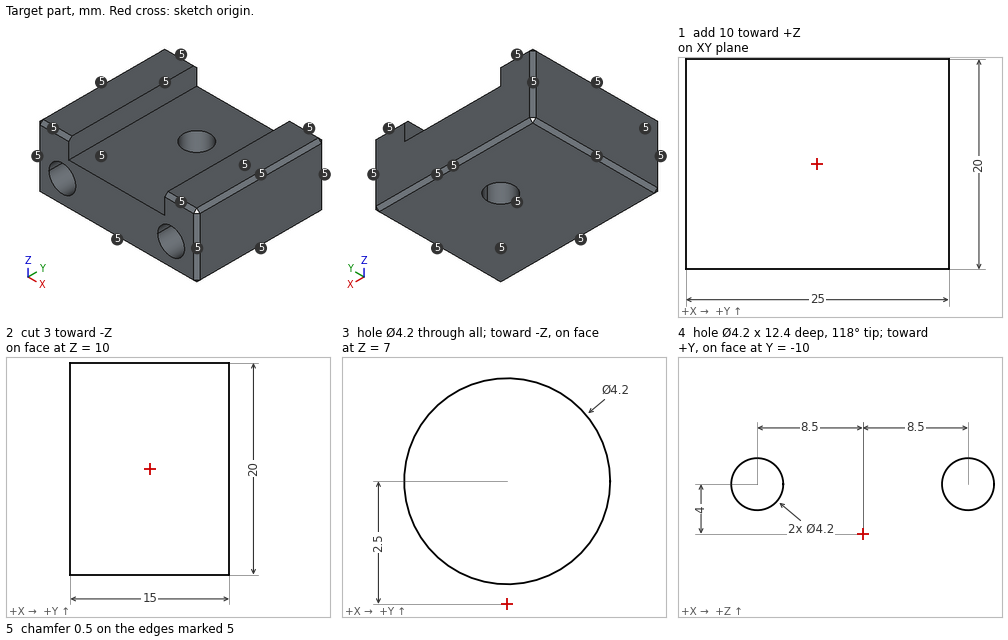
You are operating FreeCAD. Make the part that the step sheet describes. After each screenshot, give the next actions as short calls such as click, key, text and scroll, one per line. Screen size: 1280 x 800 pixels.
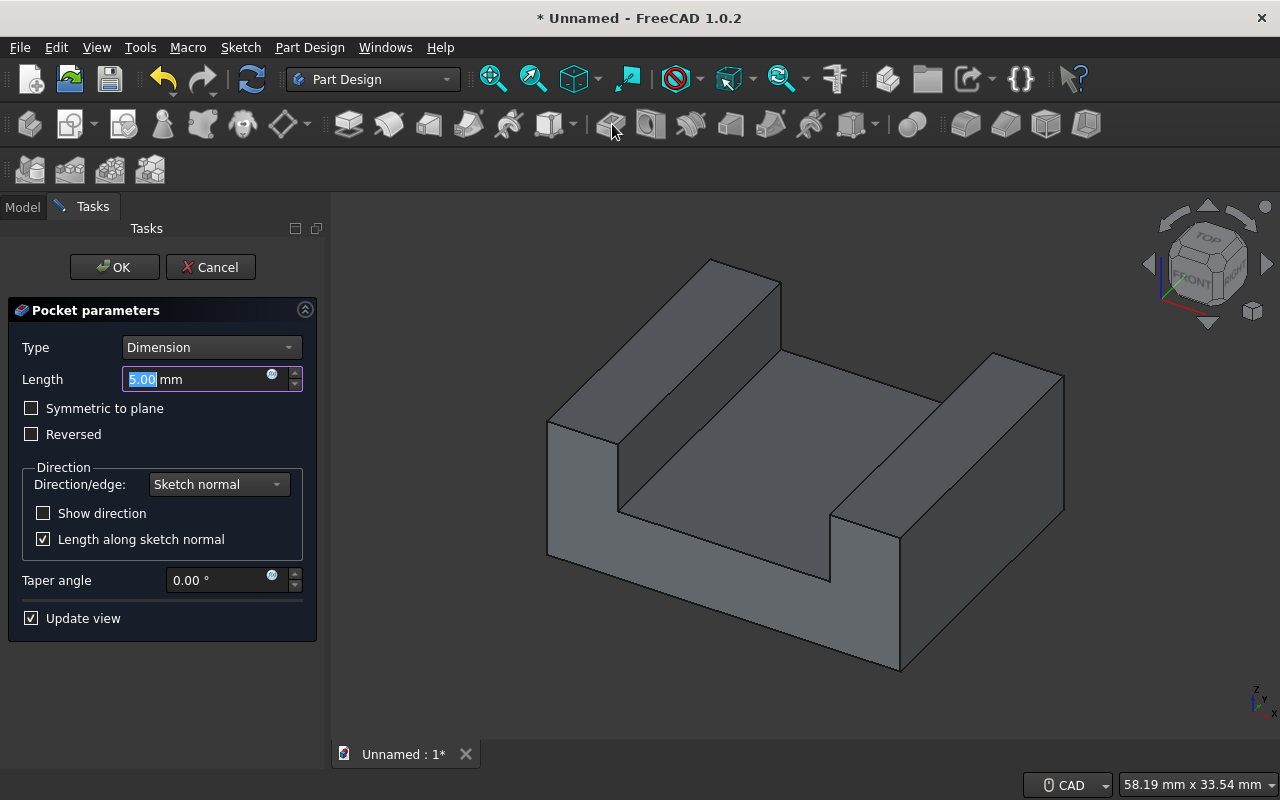
text(3)
key(Tab)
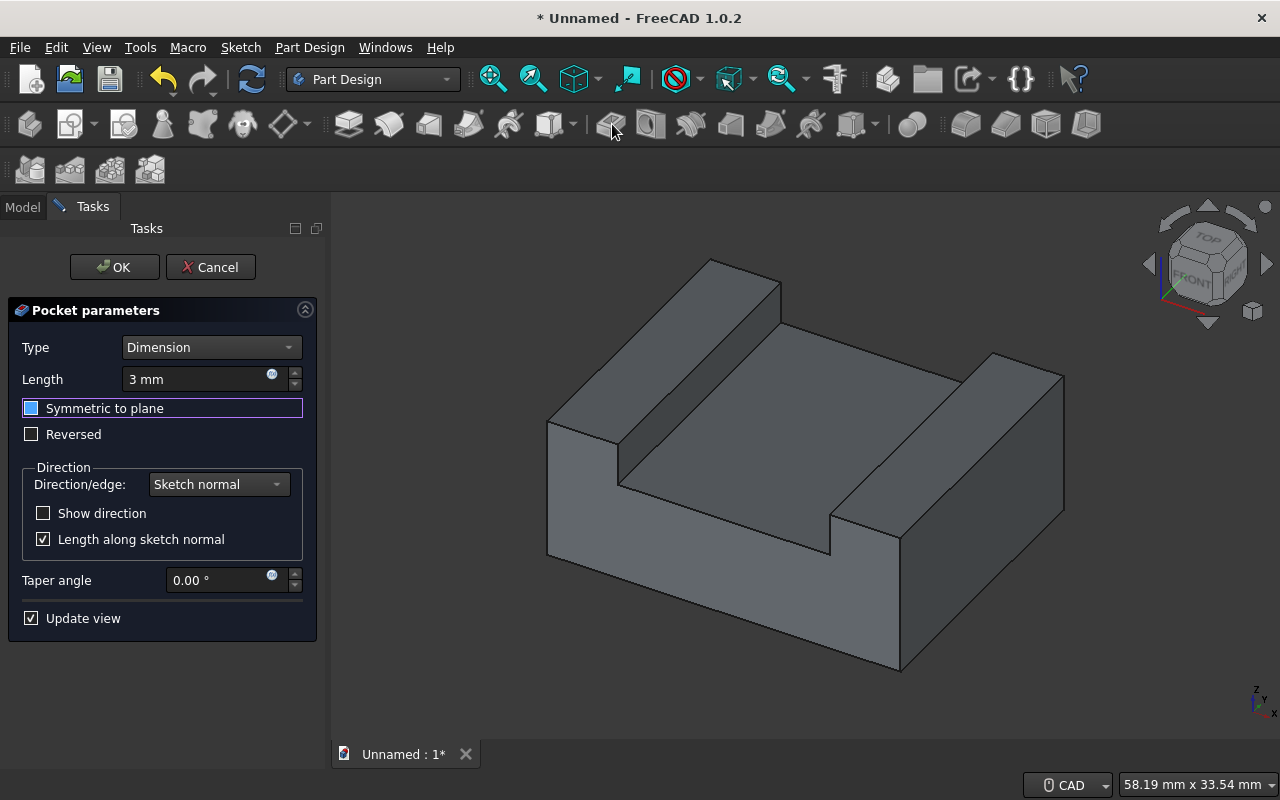
click(115, 267)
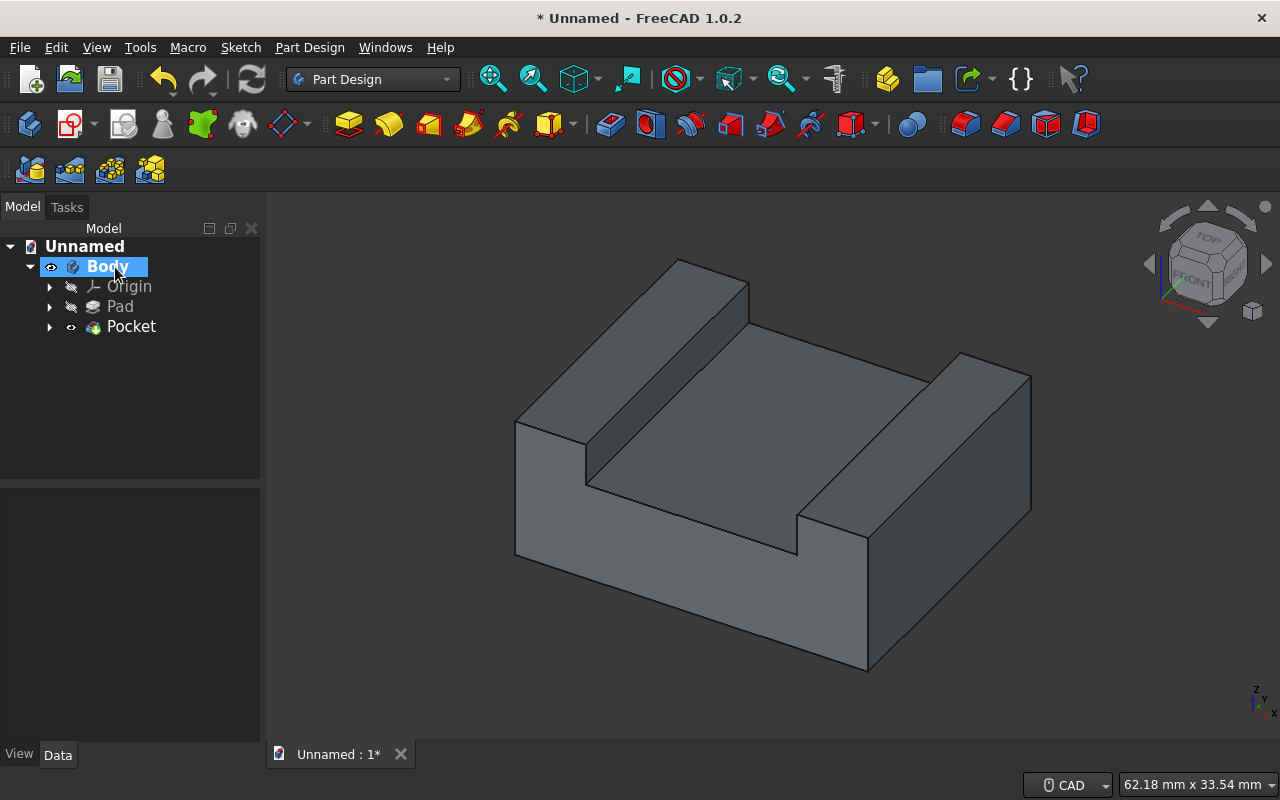
click(773, 438)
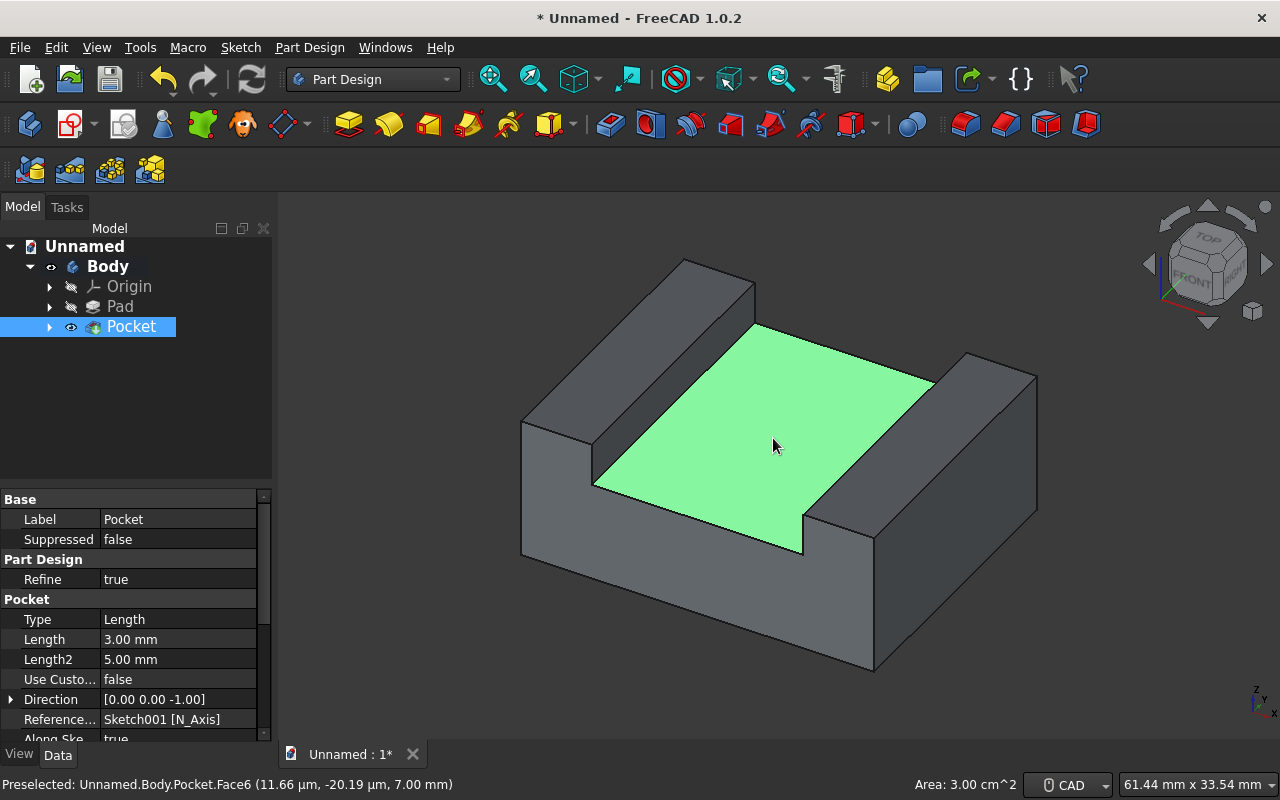
click(70, 124)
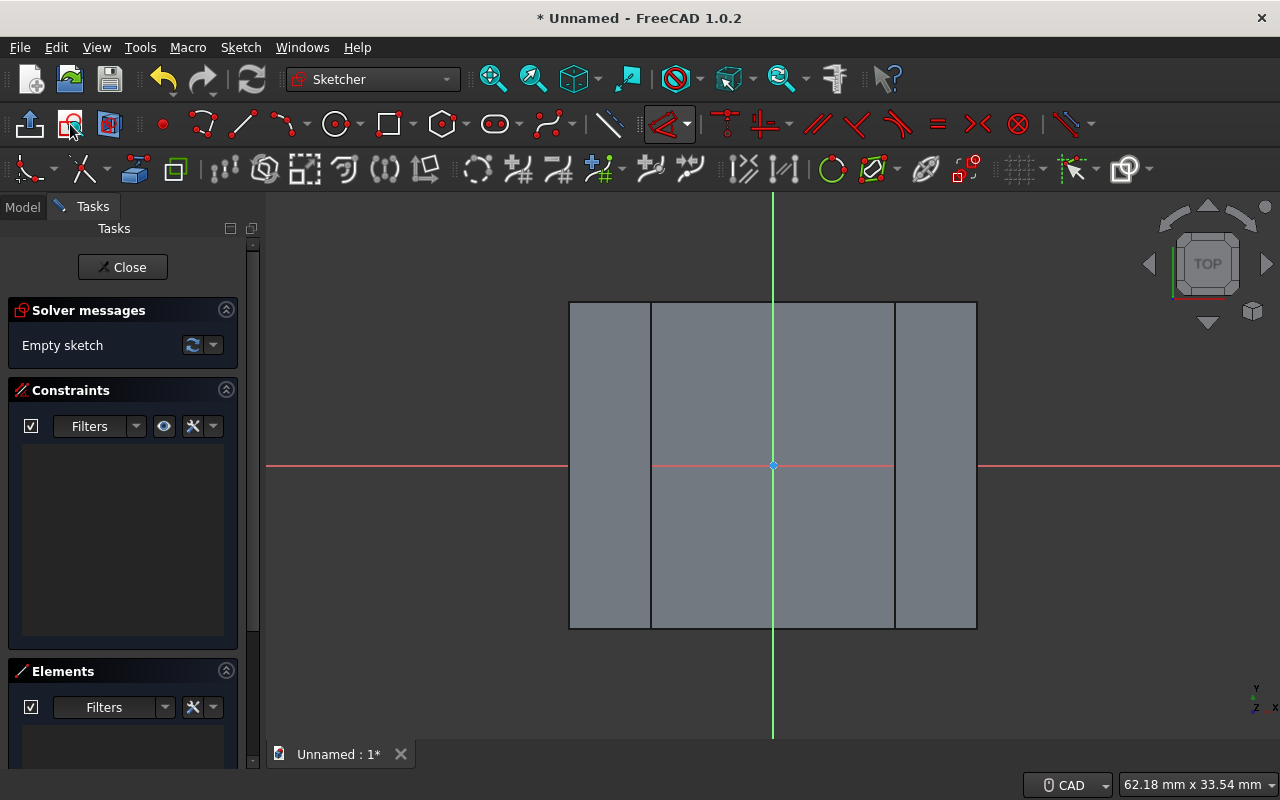
key(q)
key(s)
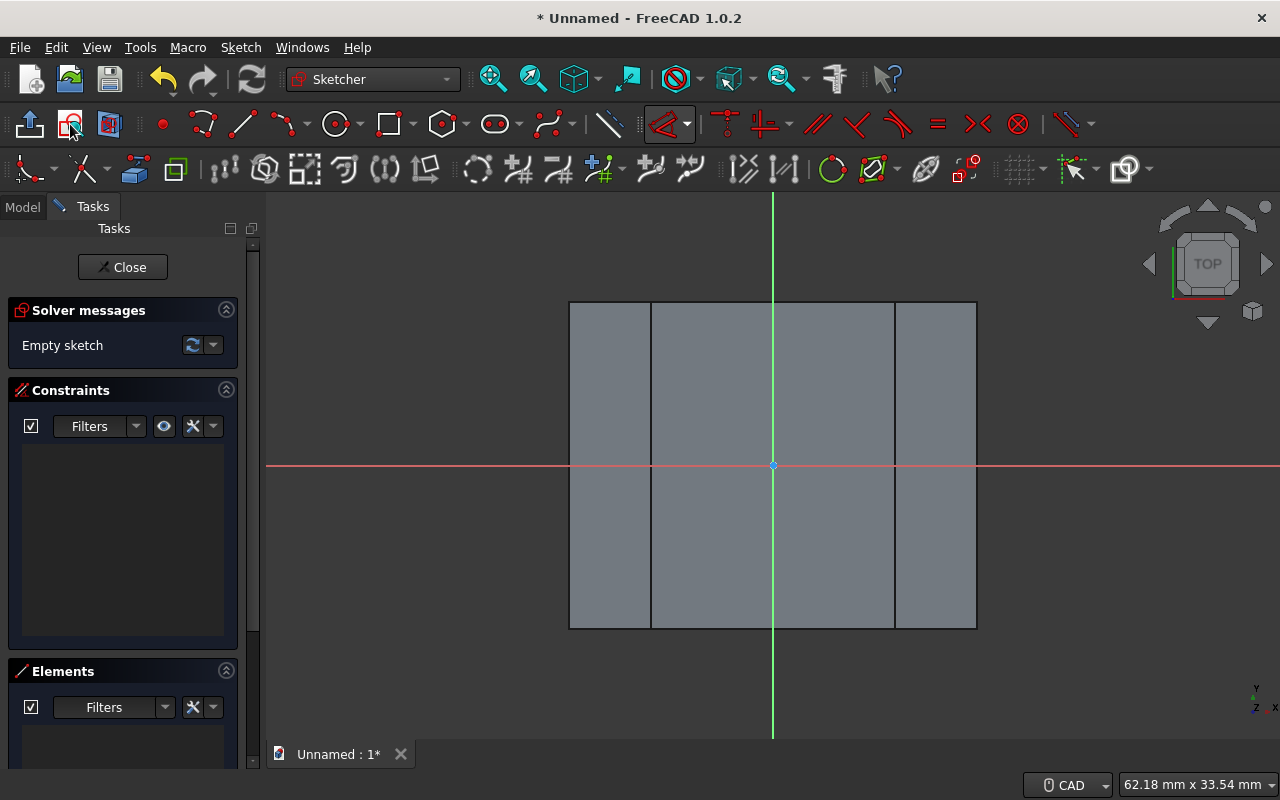
scroll(790, 419, up, 8)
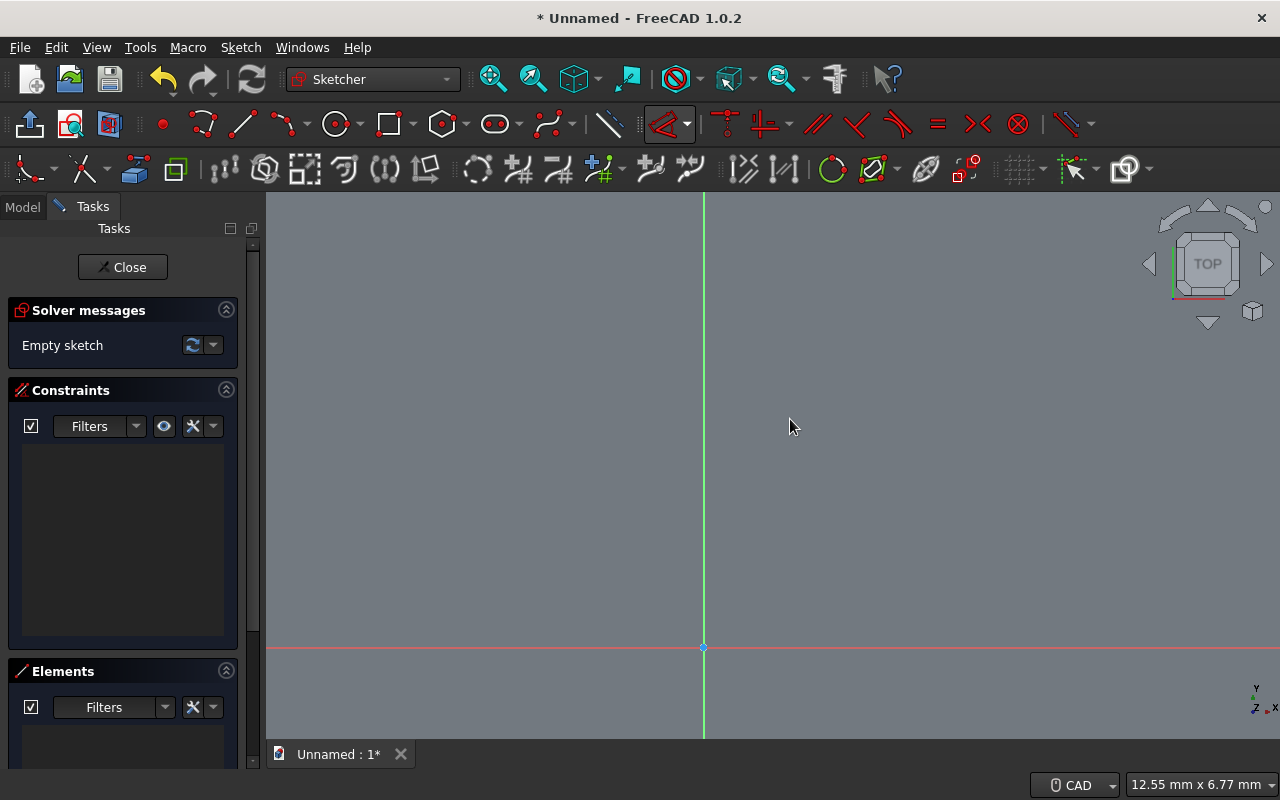
key(g)
key(c)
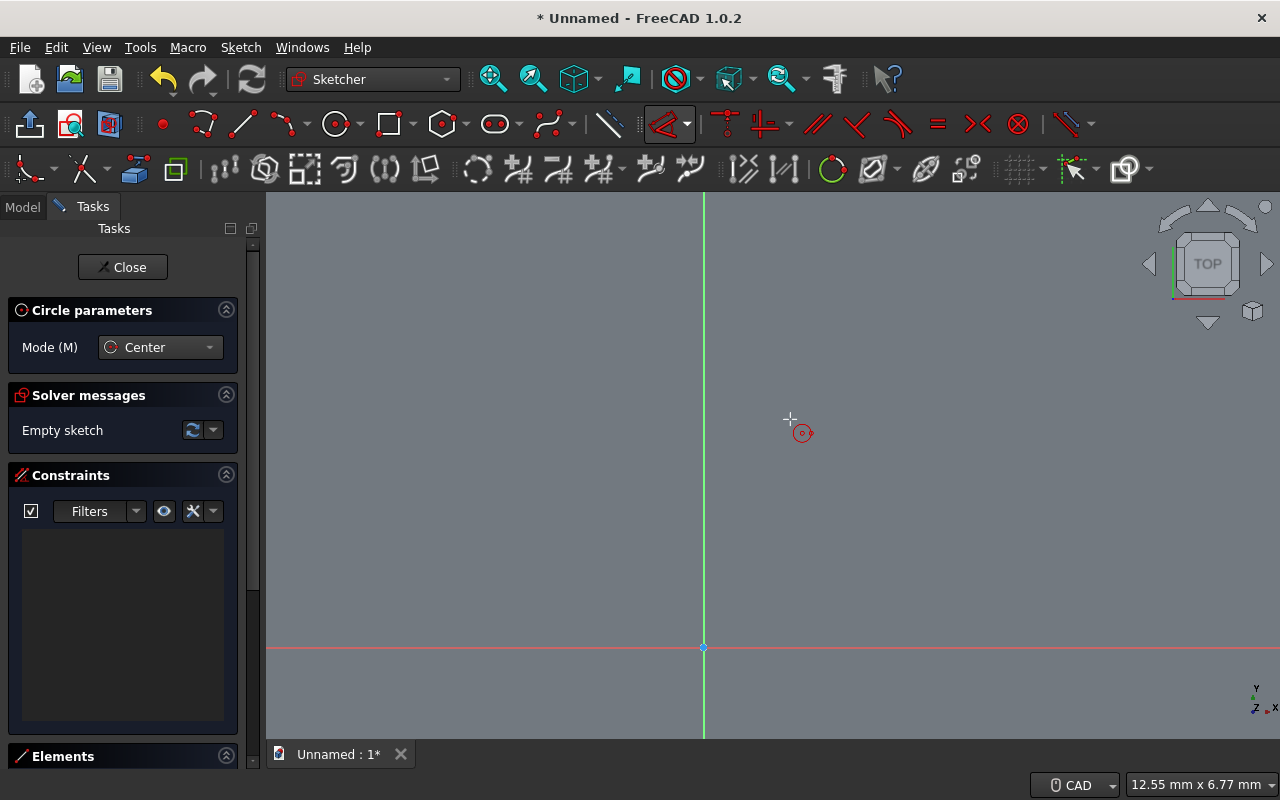
click(704, 446)
move(824, 326)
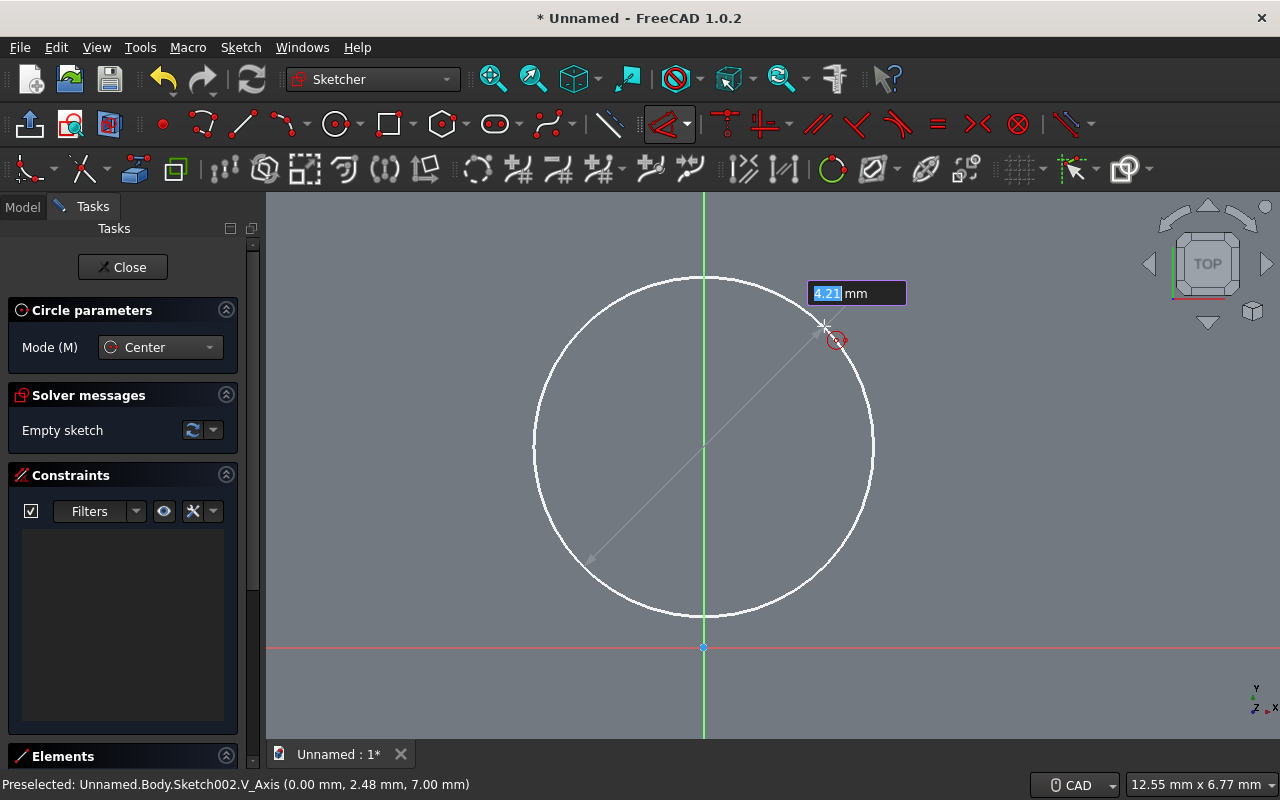
text(4.2)
key(Return)
key(Escape)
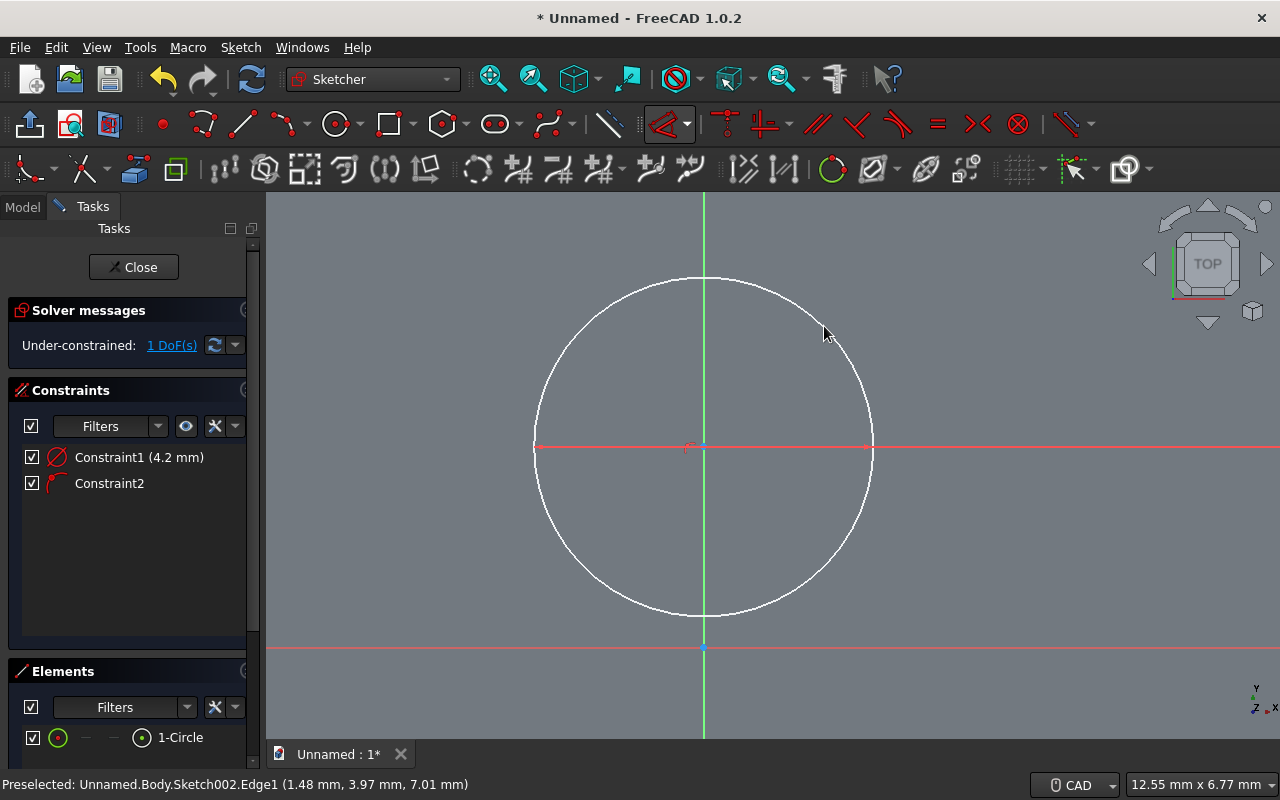
click(664, 124)